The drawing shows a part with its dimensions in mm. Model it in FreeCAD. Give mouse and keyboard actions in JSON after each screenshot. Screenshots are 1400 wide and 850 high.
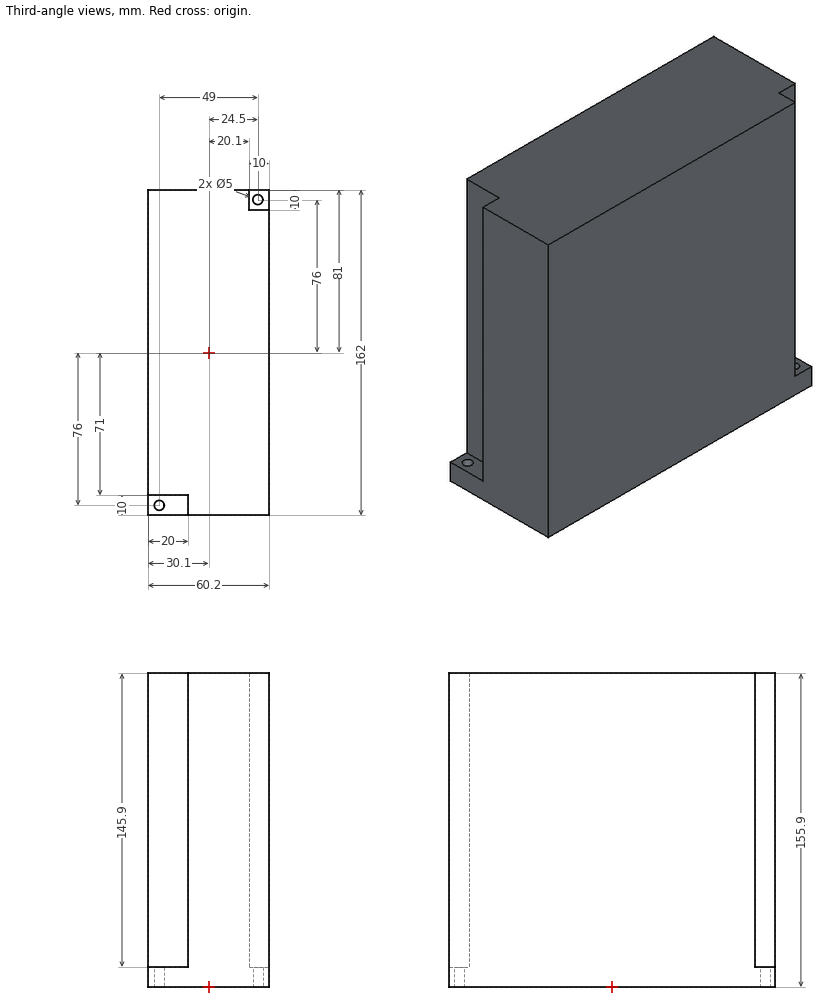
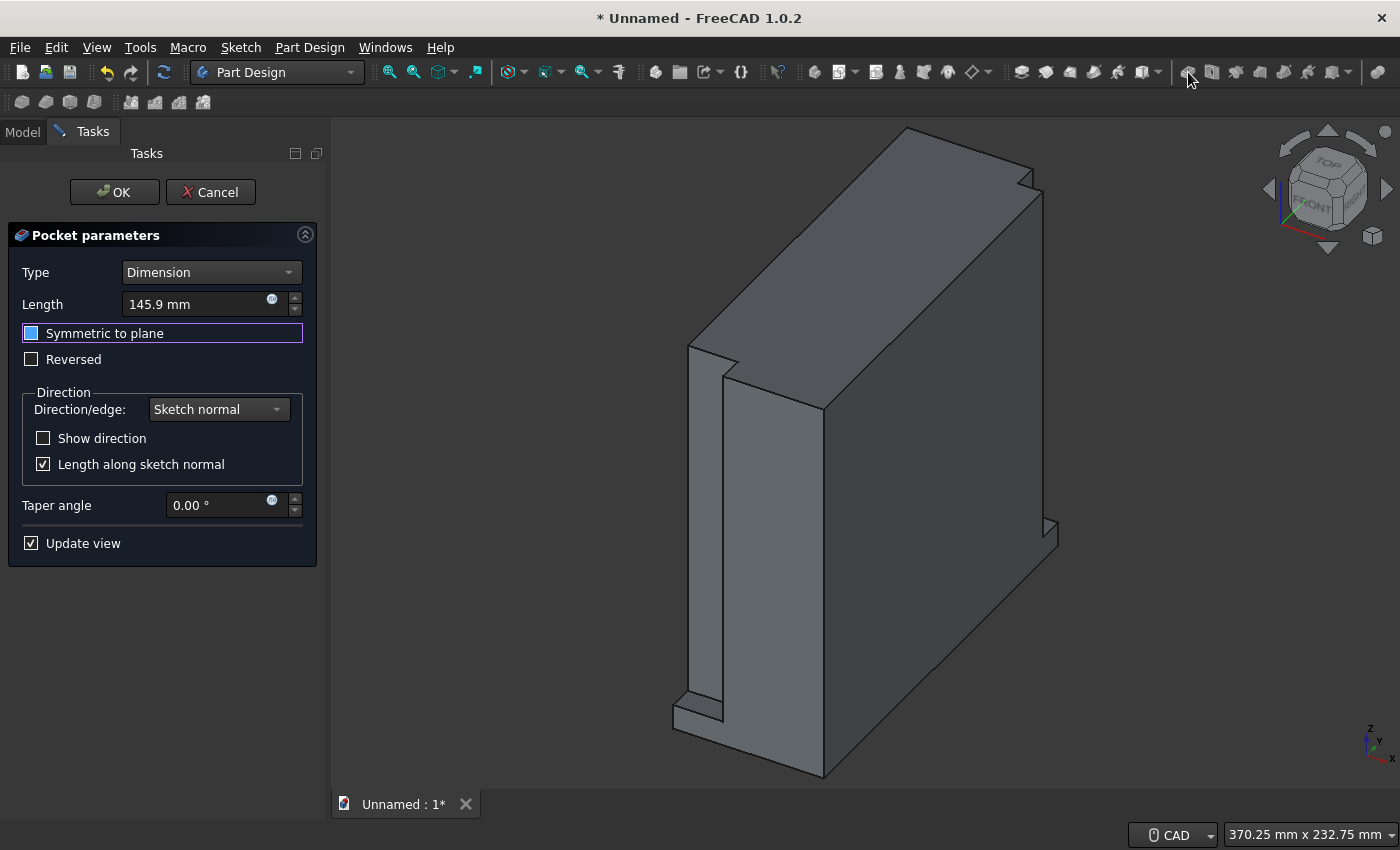
{"action": "left_click", "coordinate": [115, 192]}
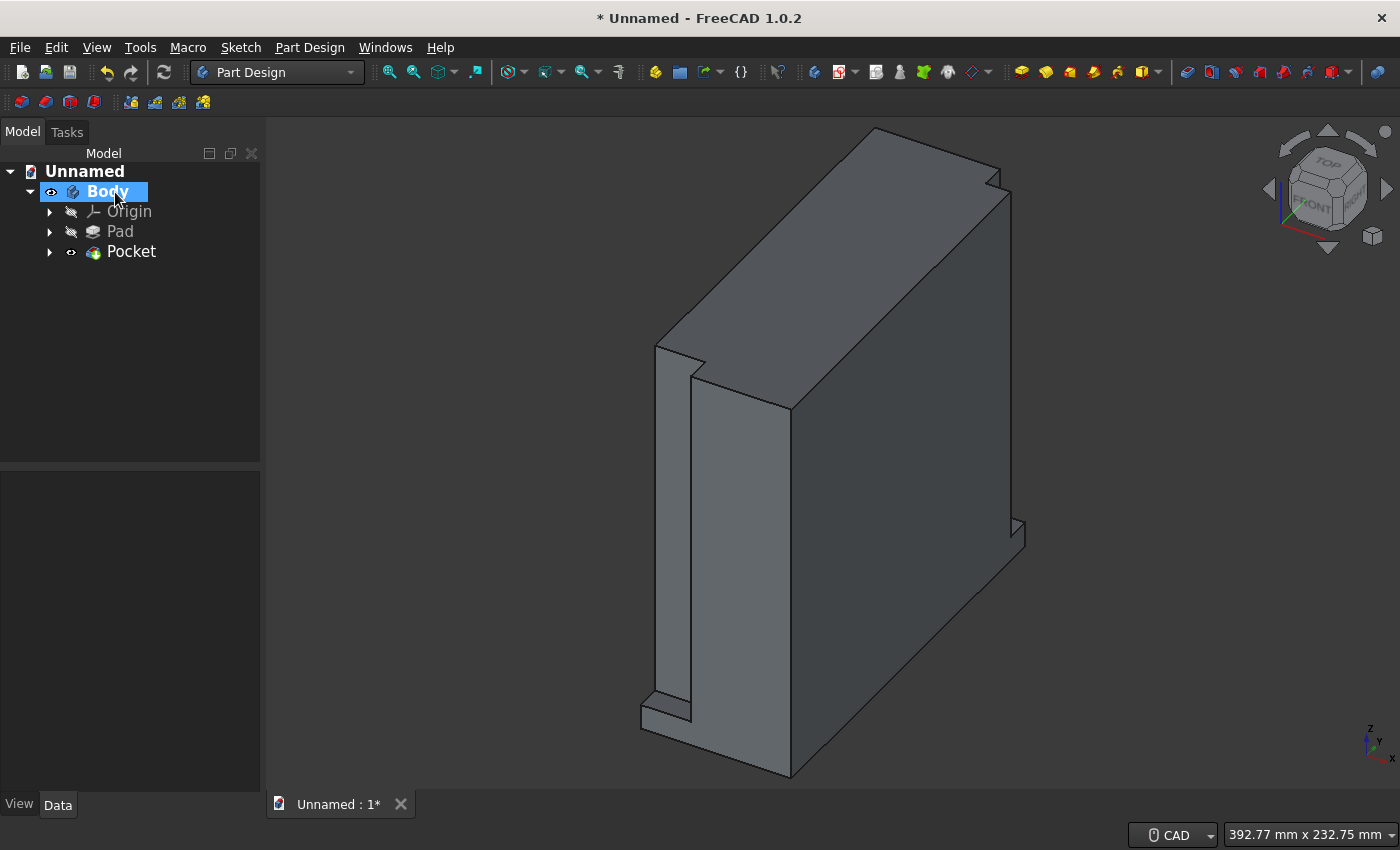
{"action": "left_click", "coordinate": [900, 201]}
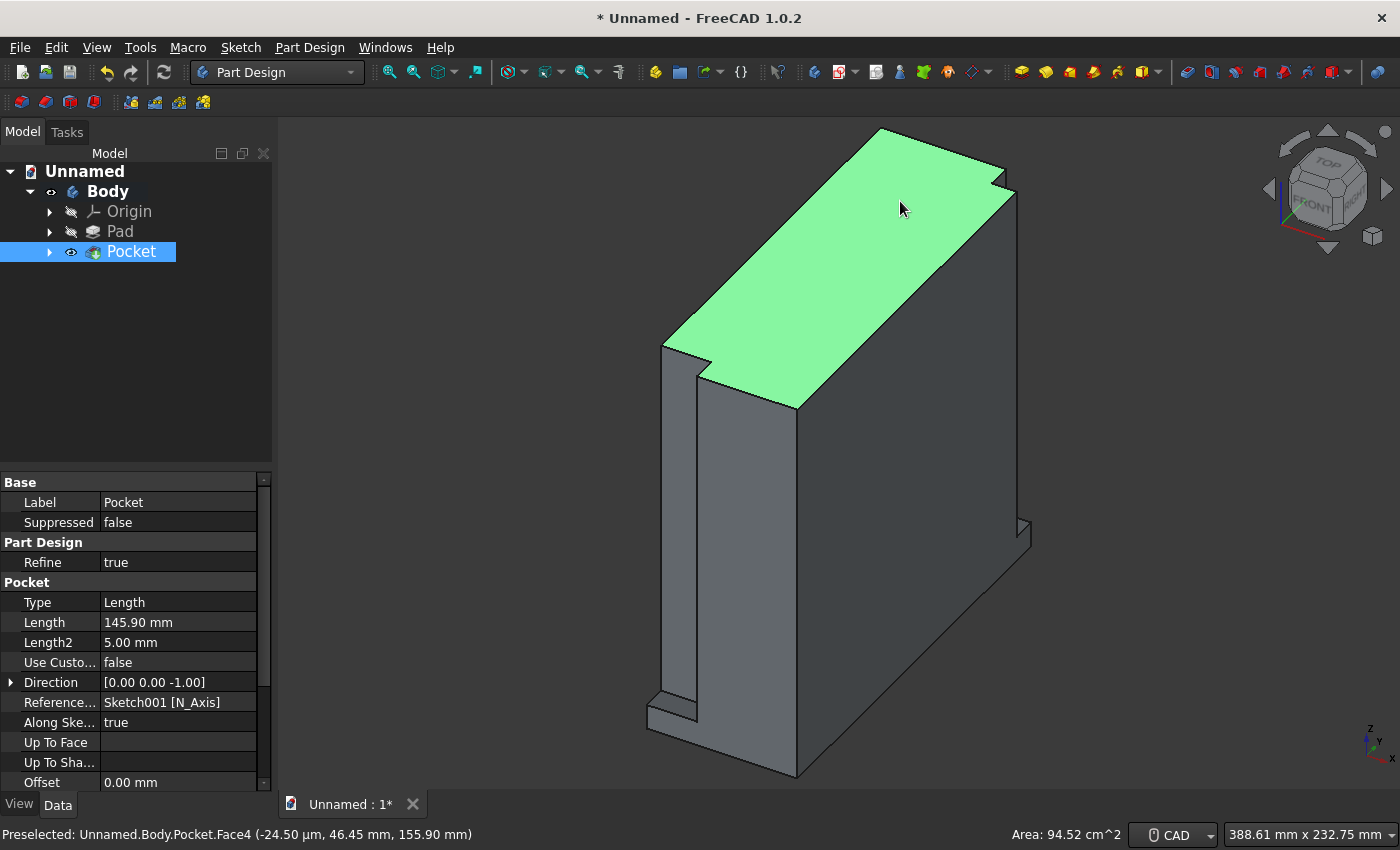
{"action": "left_click", "coordinate": [840, 72]}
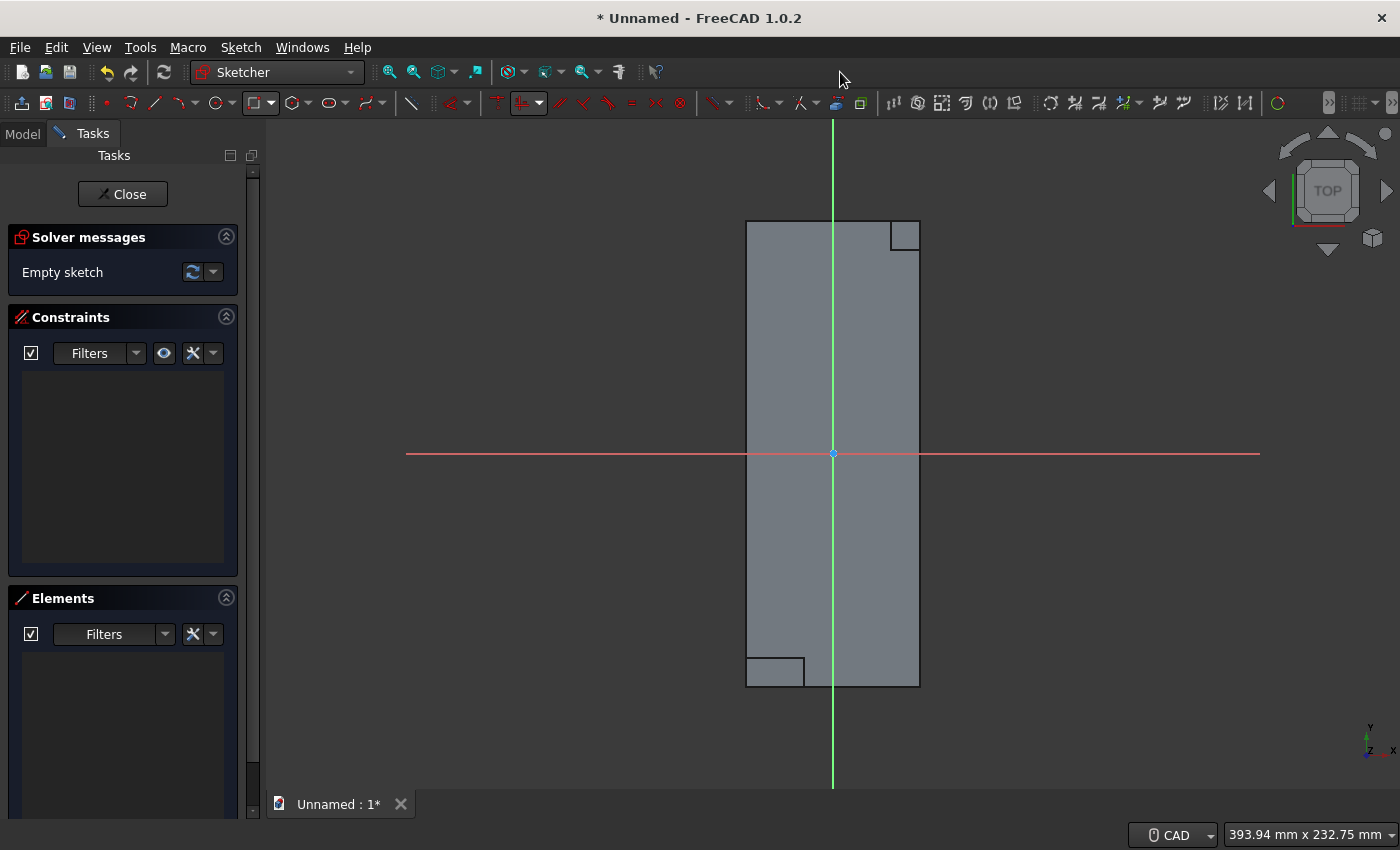
{"action": "left_click", "coordinate": [216, 104]}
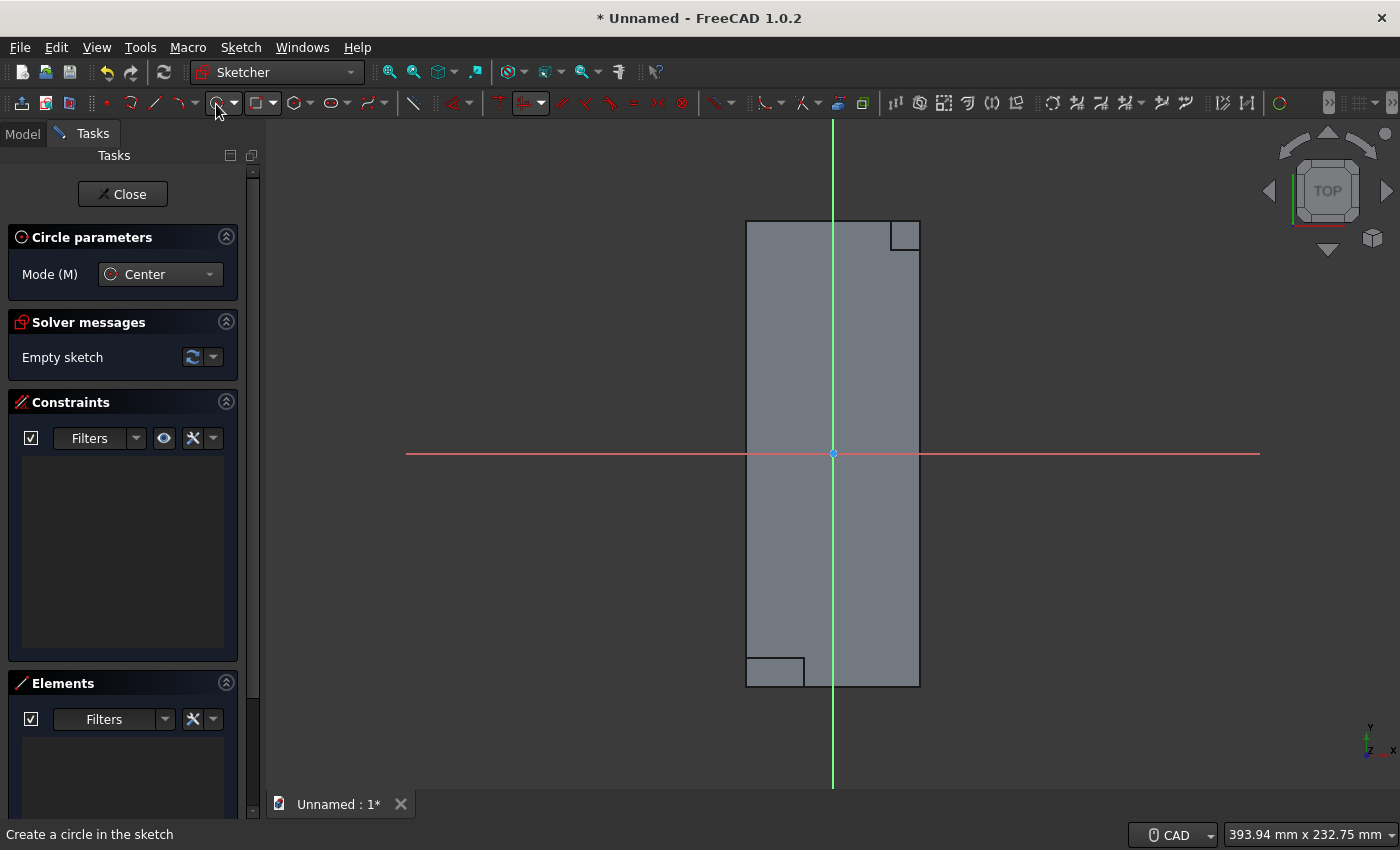
{"action": "scroll", "coordinate": [904, 235], "scroll_direction": "up", "scroll_amount": 6}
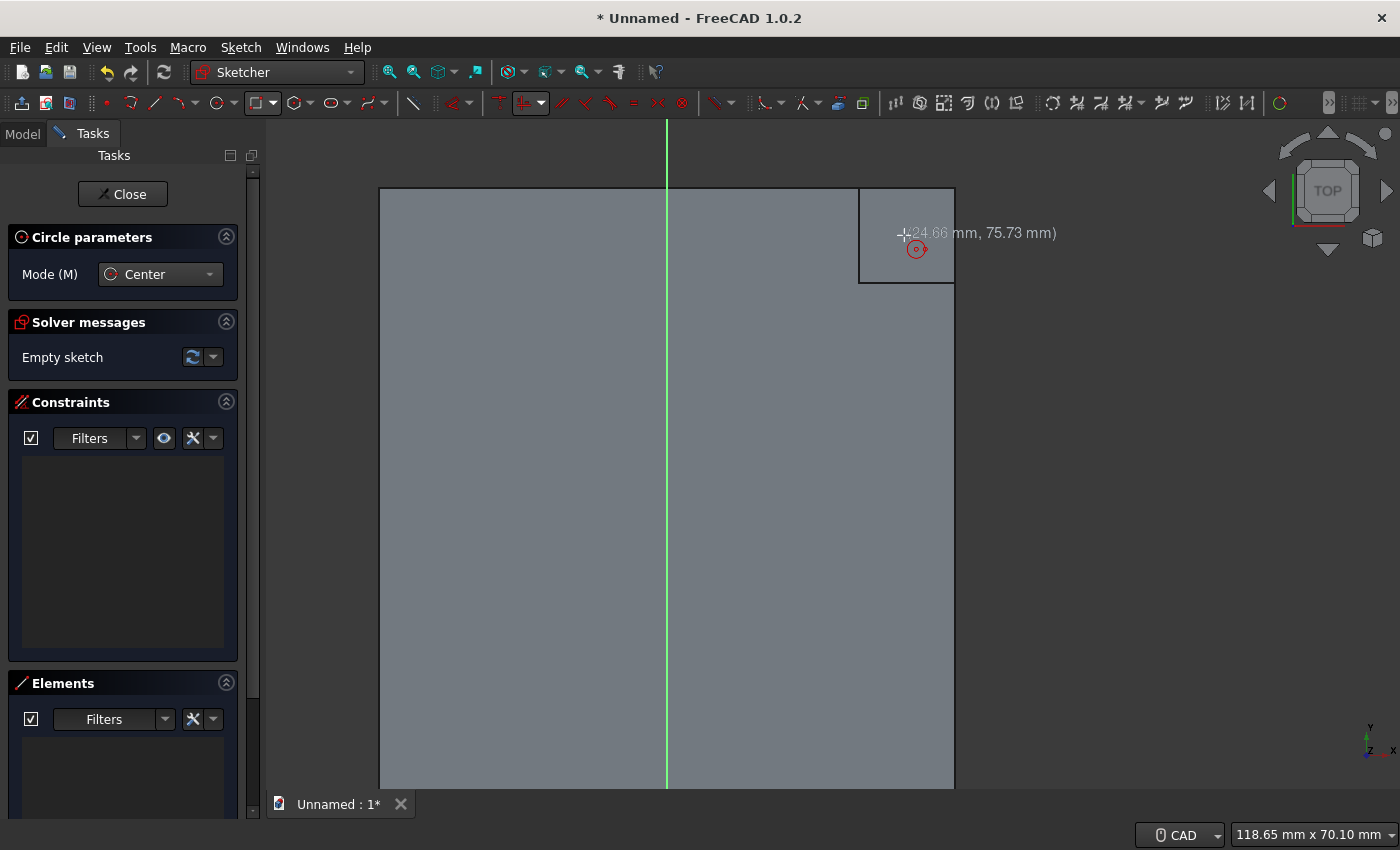
{"action": "left_click", "coordinate": [901, 235]}
{"action": "left_click", "coordinate": [918, 218]}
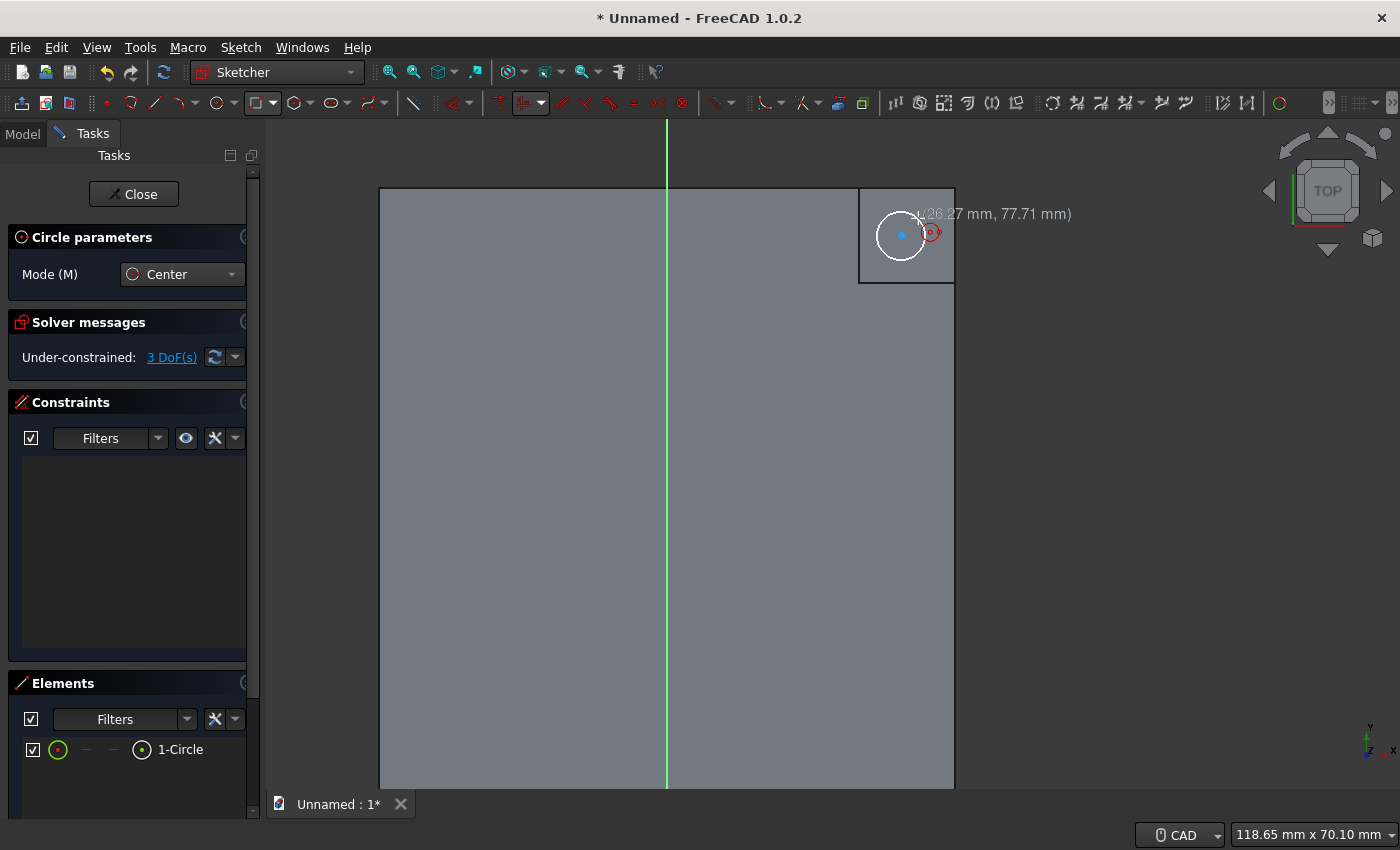
{"action": "scroll", "coordinate": [807, 235], "scroll_direction": "down", "scroll_amount": 6}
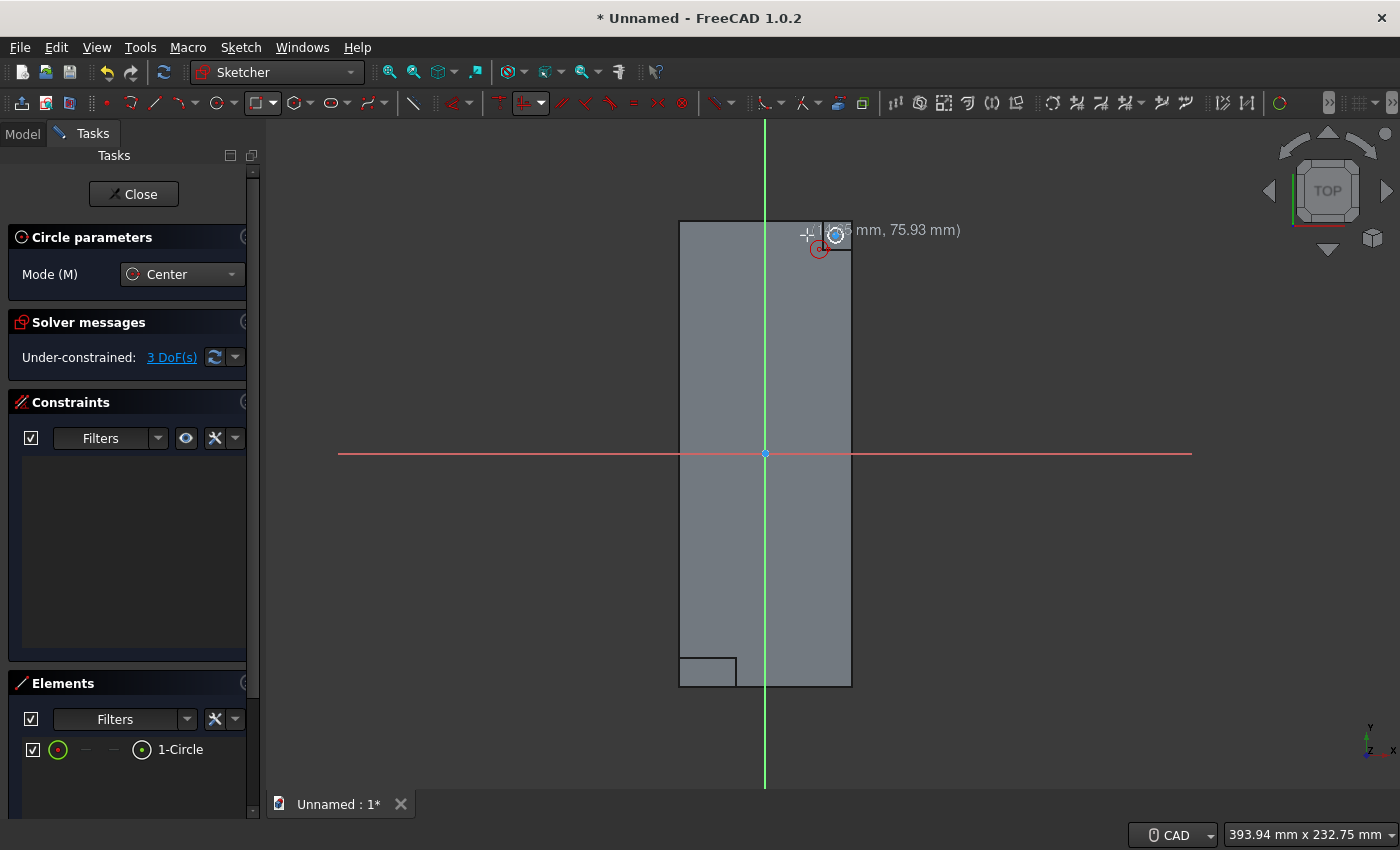
{"action": "scroll", "coordinate": [695, 673], "scroll_direction": "up", "scroll_amount": 6}